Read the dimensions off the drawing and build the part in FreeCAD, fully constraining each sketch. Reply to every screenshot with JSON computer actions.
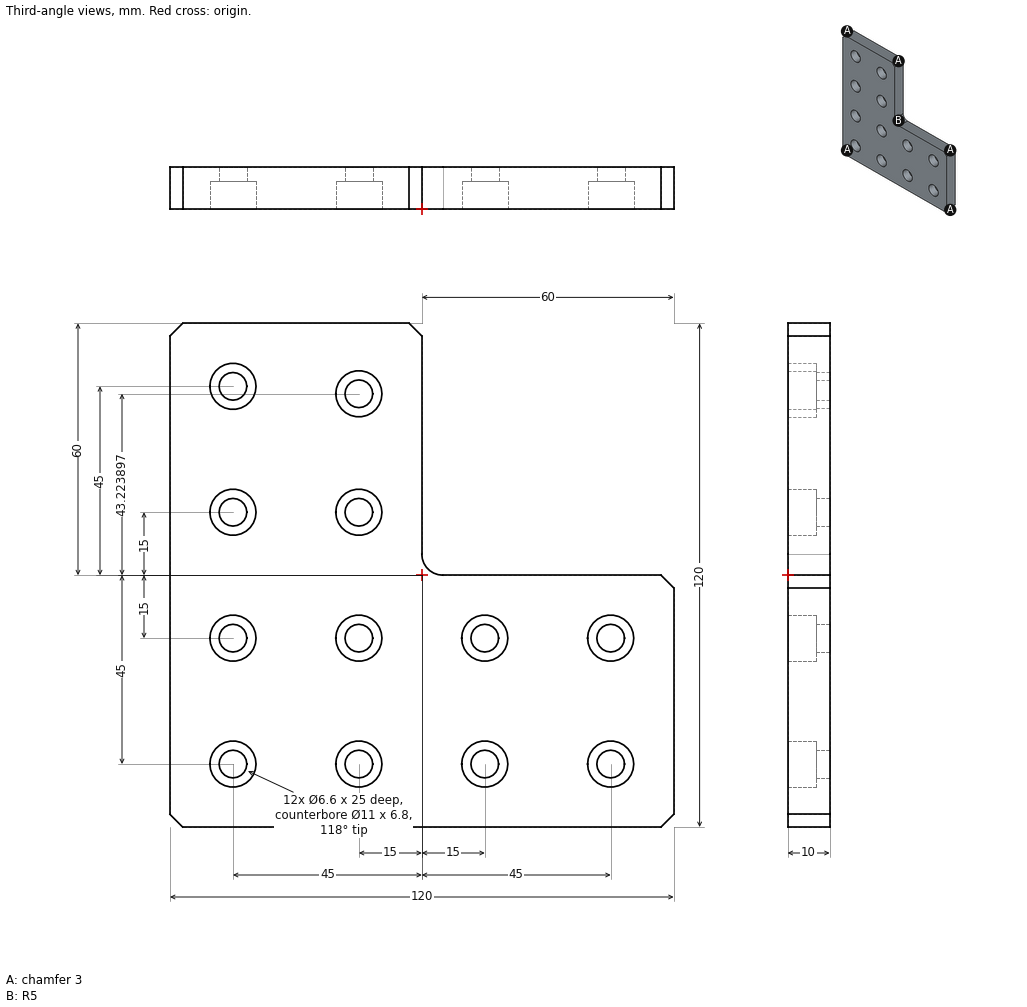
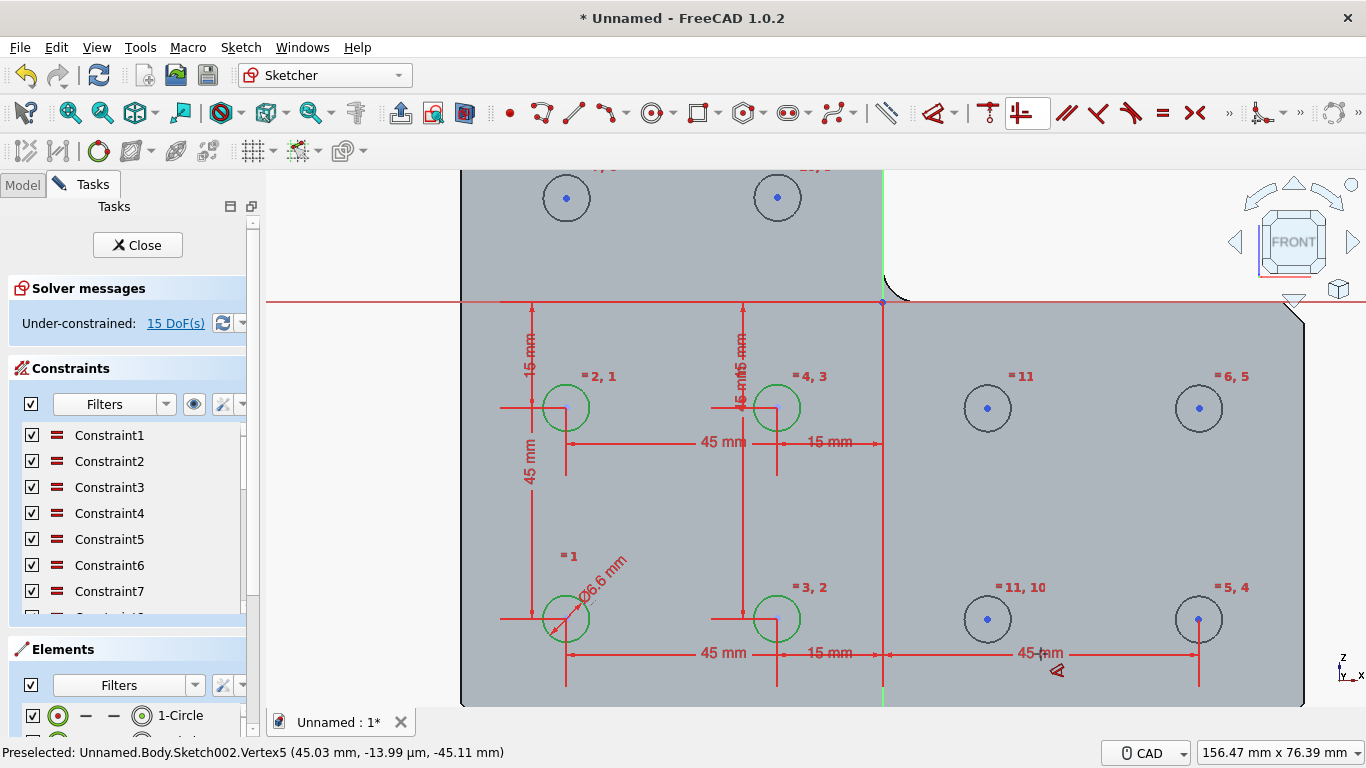
{"action": "left_click", "coordinate": [1199, 620]}
{"action": "left_click", "coordinate": [849, 388]}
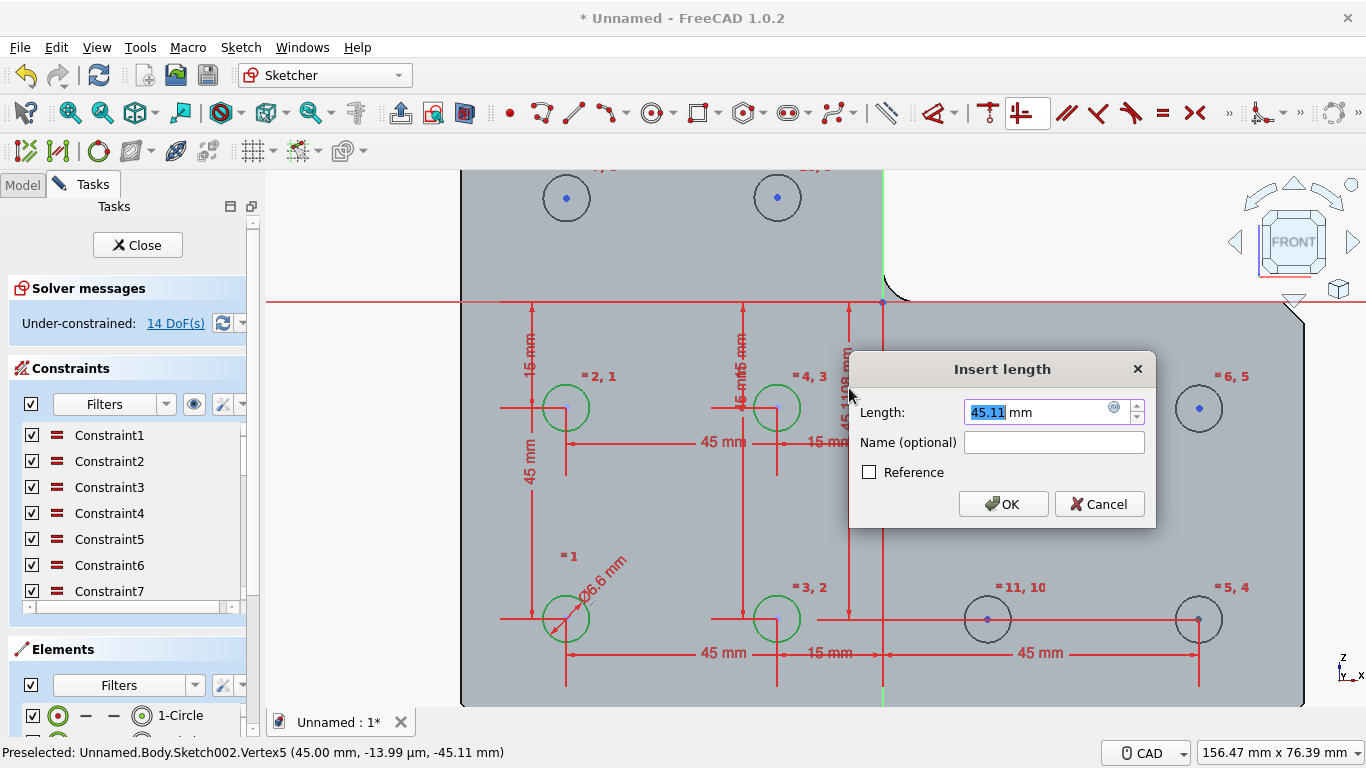
{"action": "type", "text": "45"}
{"action": "key", "text": "Return"}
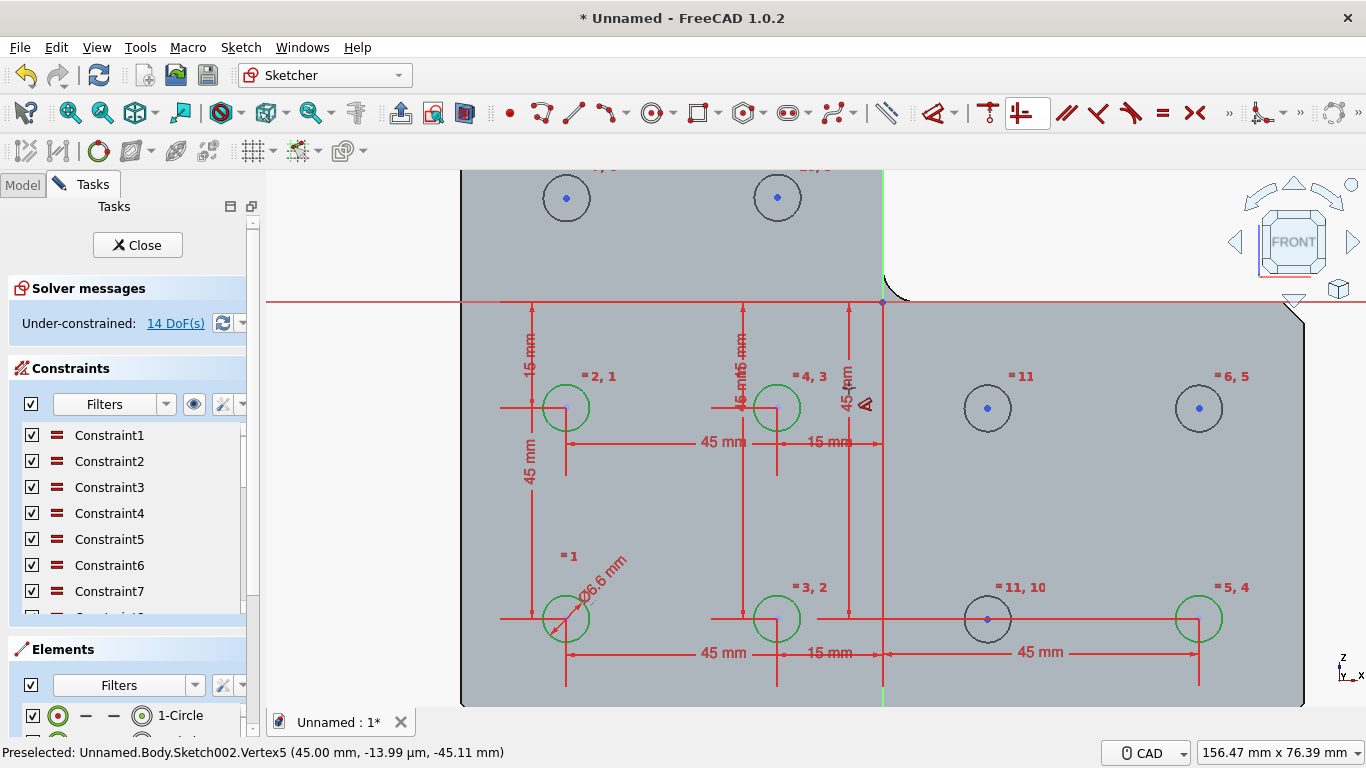
{"action": "left_click", "coordinate": [1199, 409]}
{"action": "left_click", "coordinate": [1041, 443]}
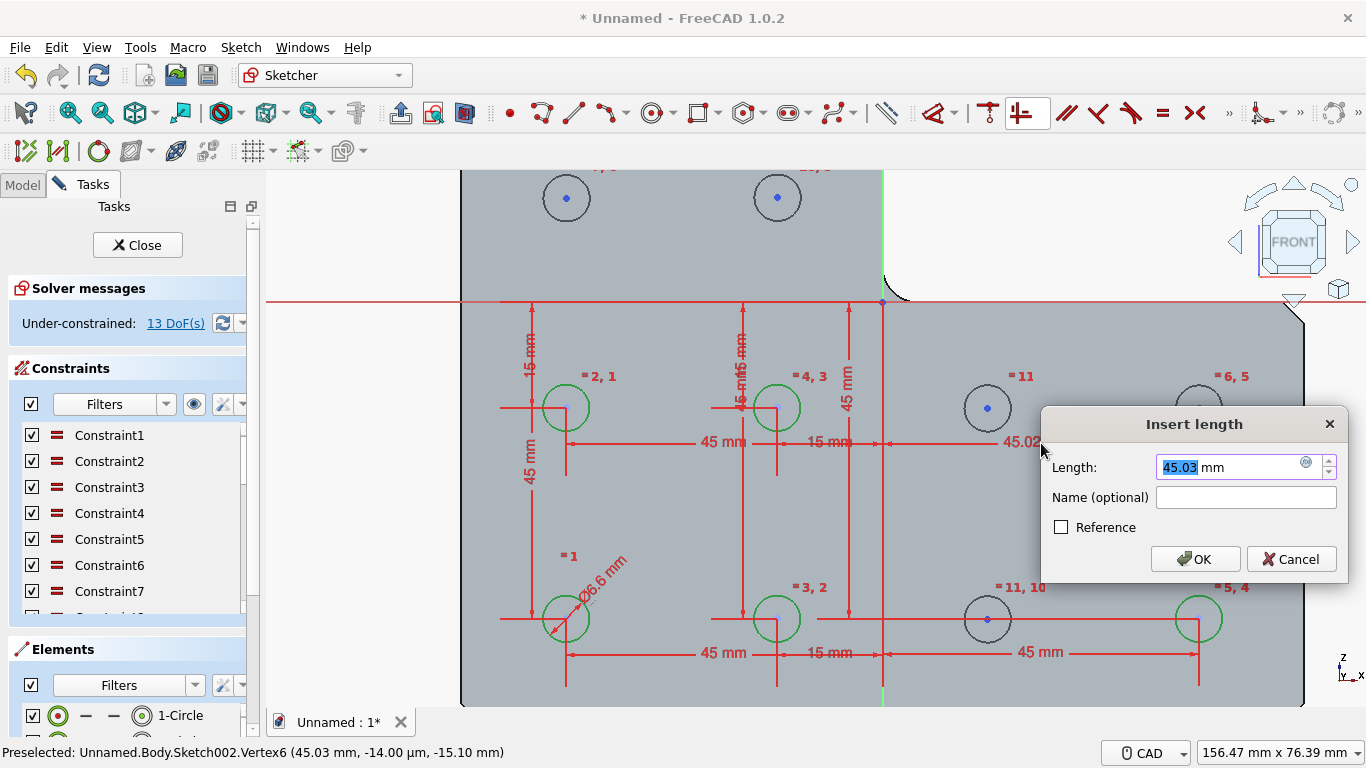
{"action": "type", "text": "45"}
{"action": "key", "text": "Return"}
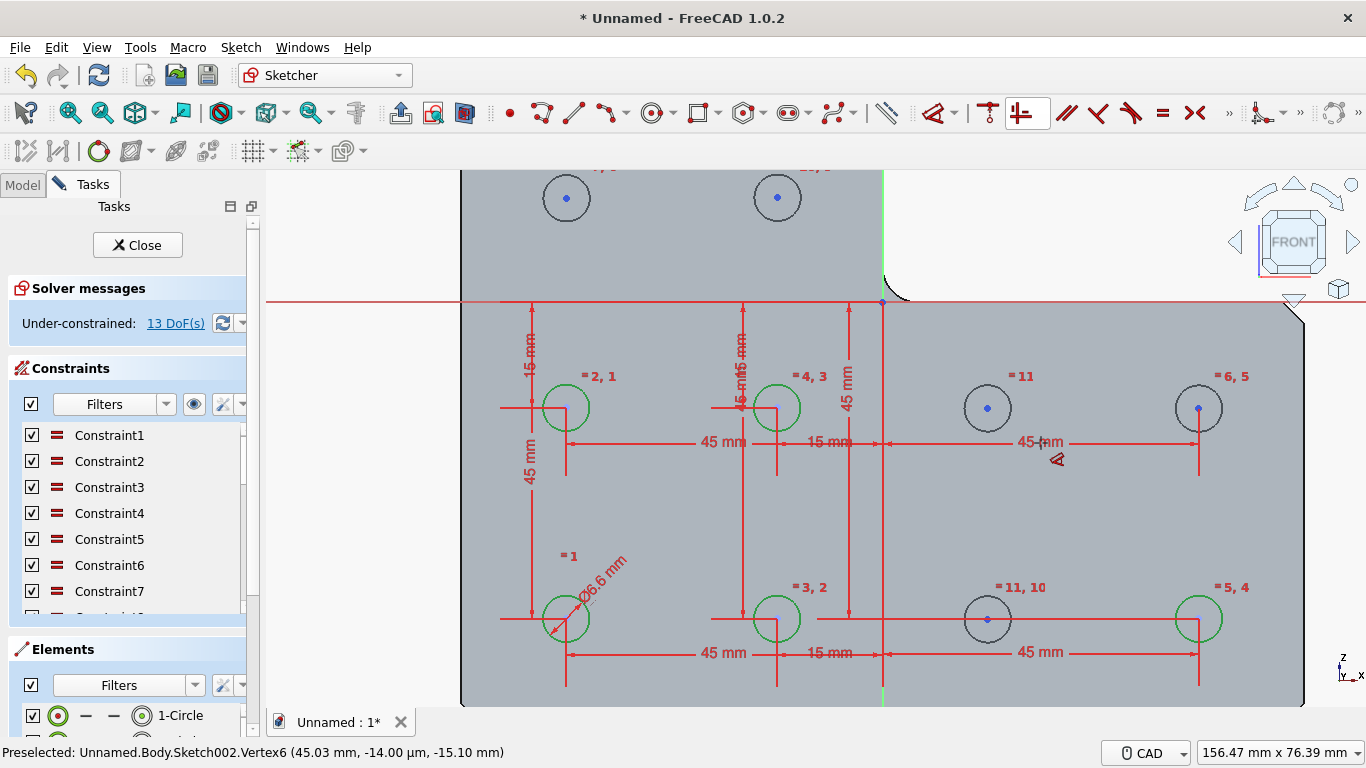
{"action": "left_click", "coordinate": [1199, 409]}
{"action": "left_click", "coordinate": [849, 356]}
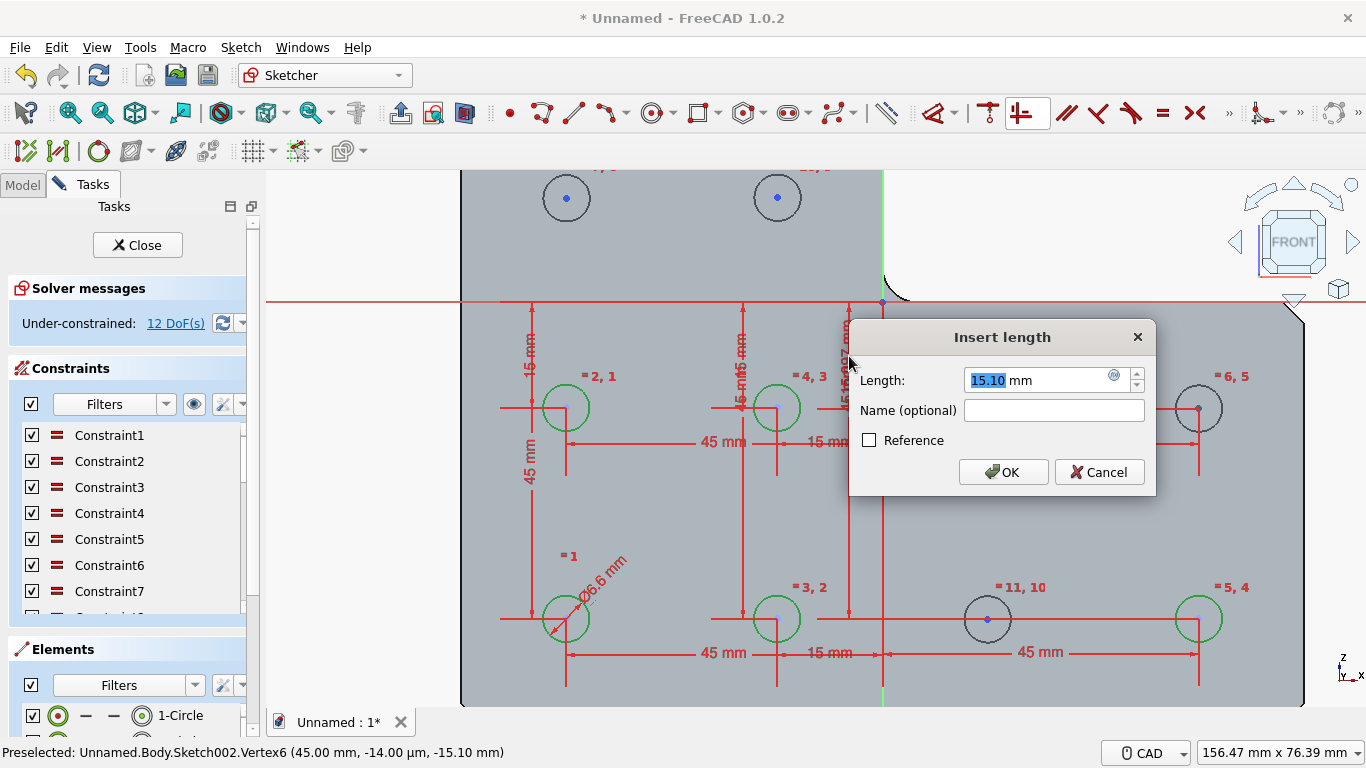
{"action": "type", "text": "15"}
{"action": "key", "text": "Return"}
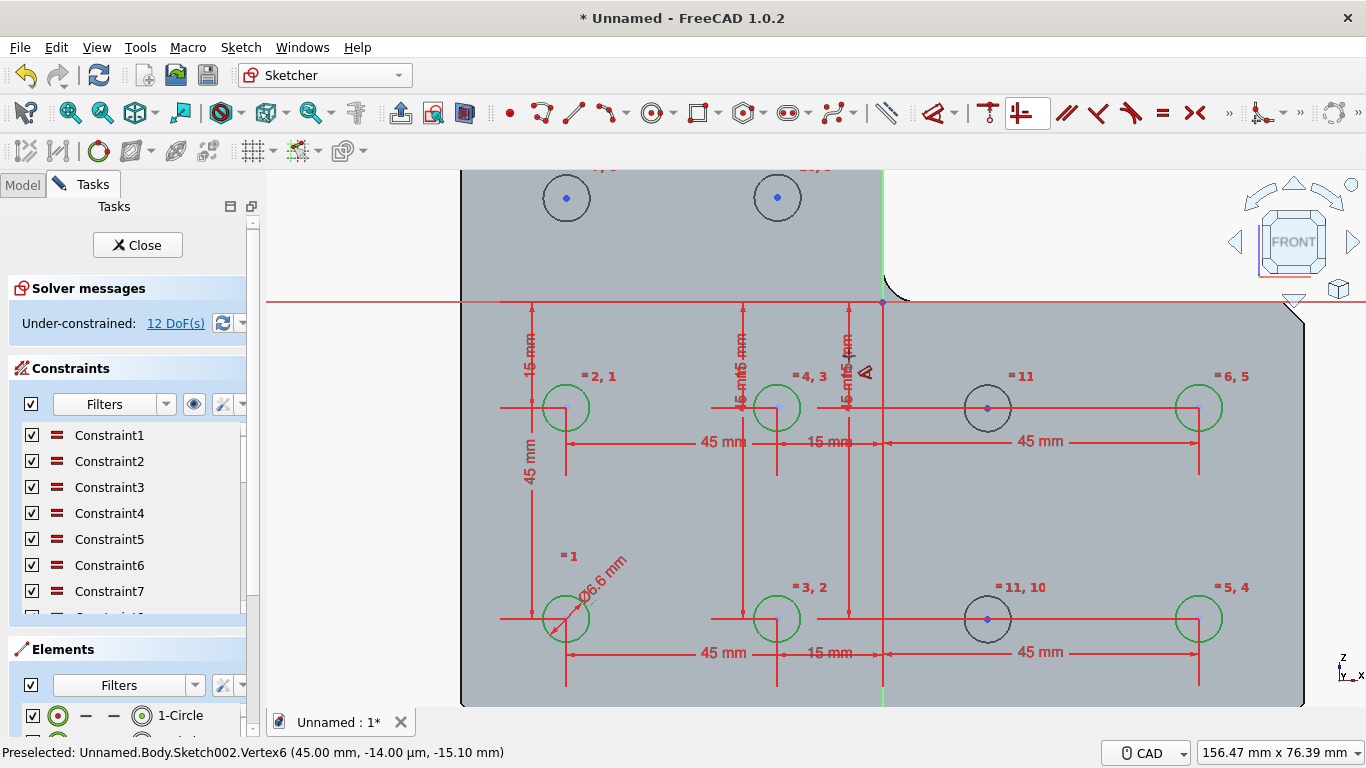
{"action": "left_click", "coordinate": [567, 198]}
{"action": "left_click", "coordinate": [652, 336]}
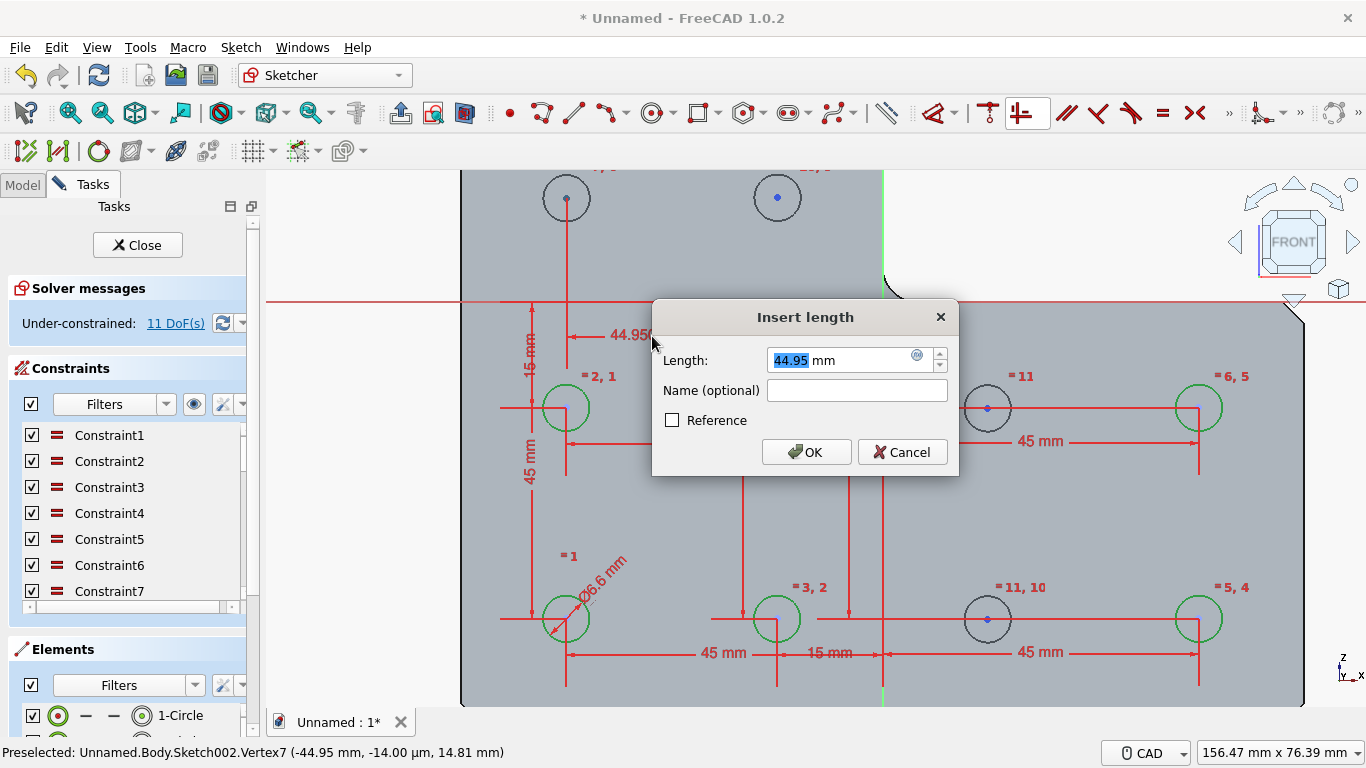
{"action": "type", "text": "45"}
{"action": "key", "text": "Return"}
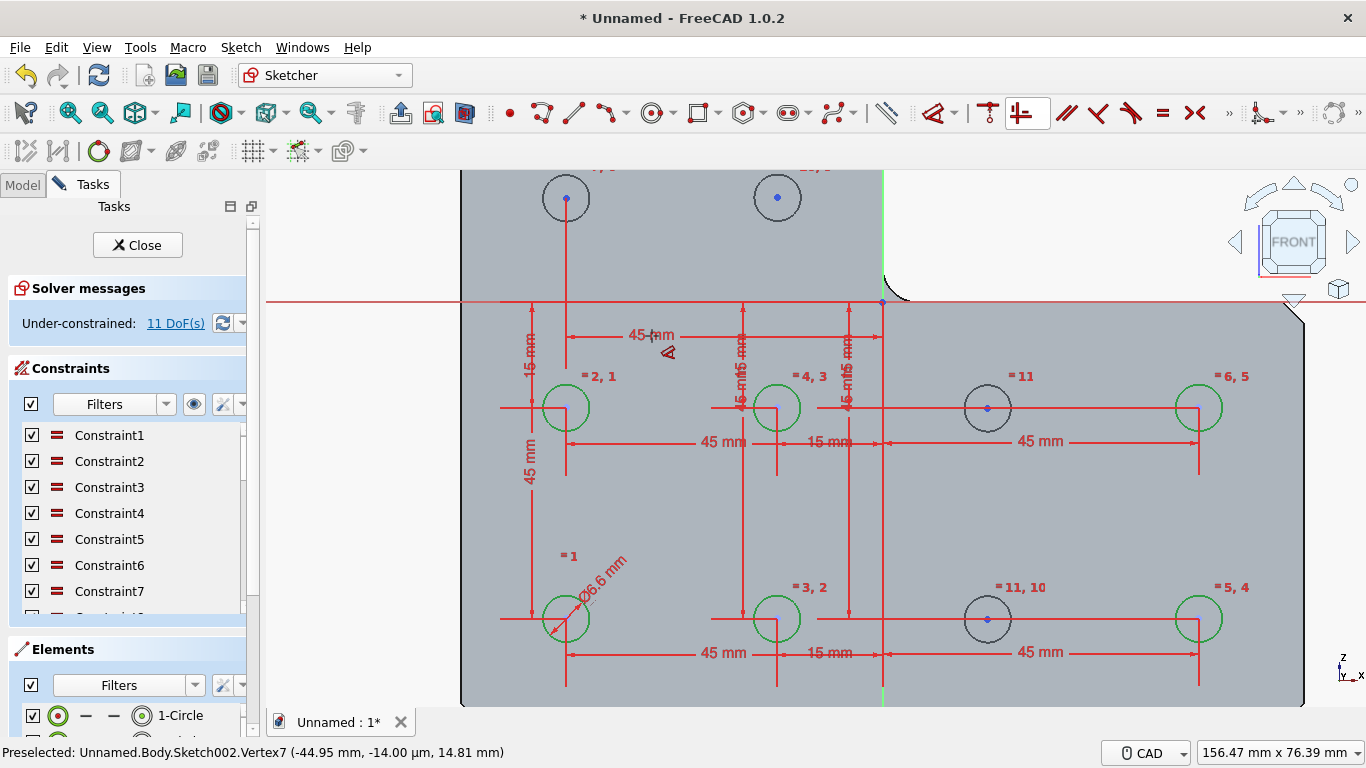
{"action": "left_click", "coordinate": [566, 198]}
{"action": "left_click", "coordinate": [532, 250]}